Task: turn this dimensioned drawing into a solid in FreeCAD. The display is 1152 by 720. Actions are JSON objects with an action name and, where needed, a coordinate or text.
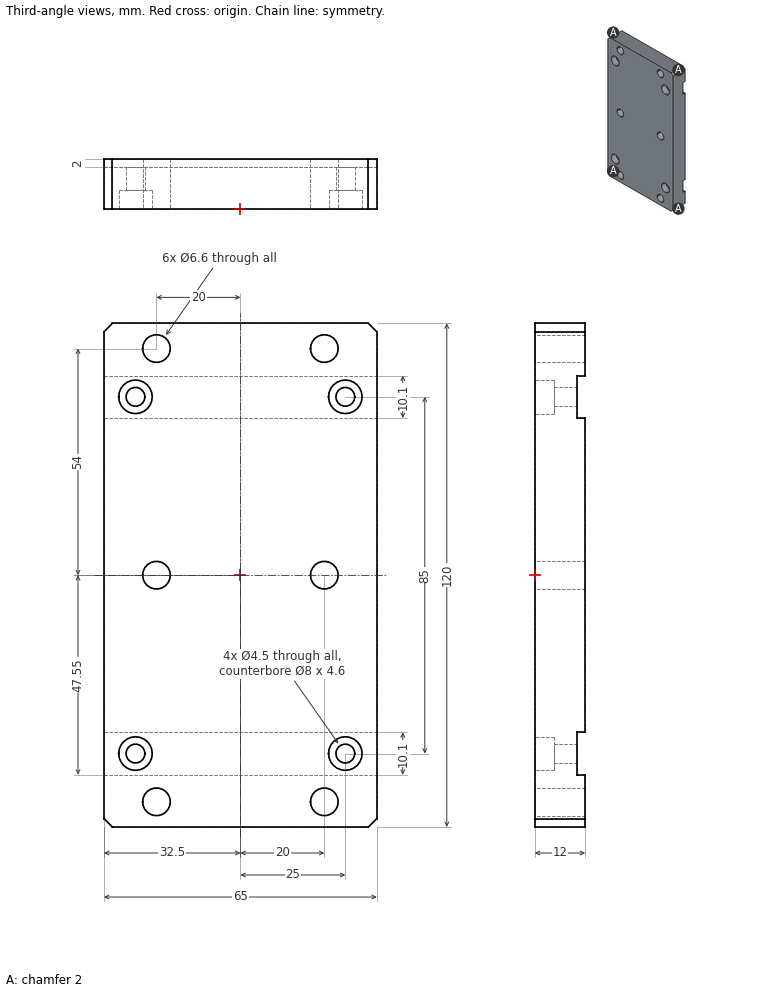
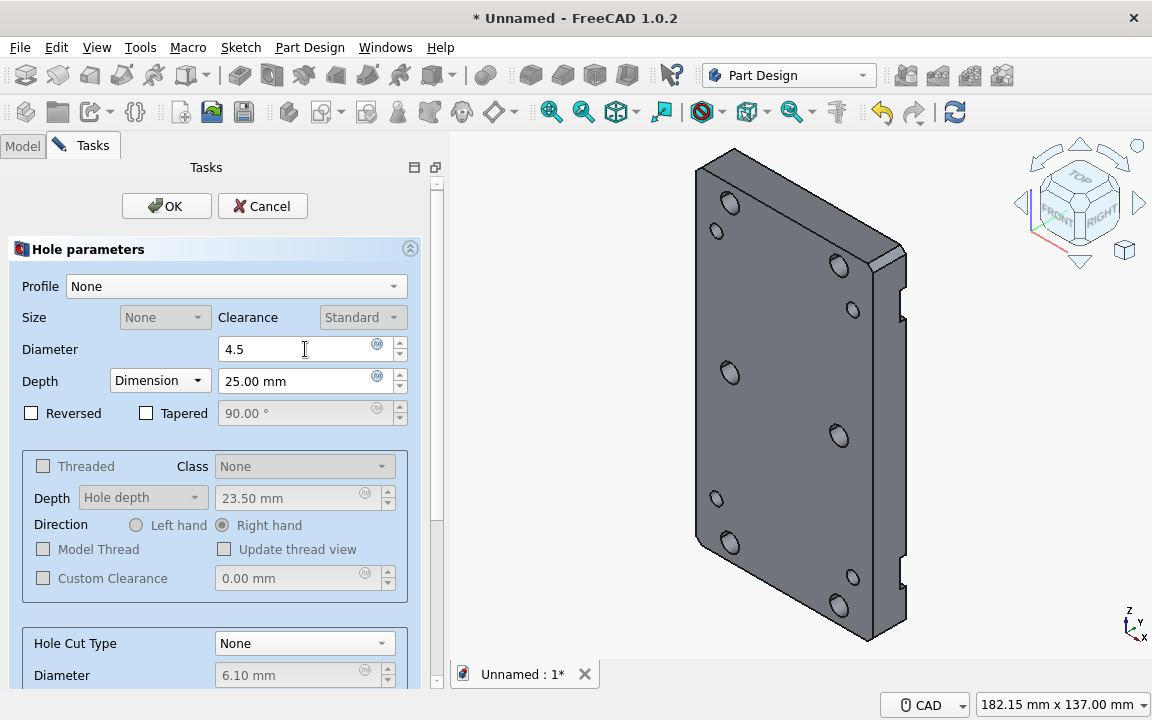
{"action": "left_click", "coordinate": [161, 380]}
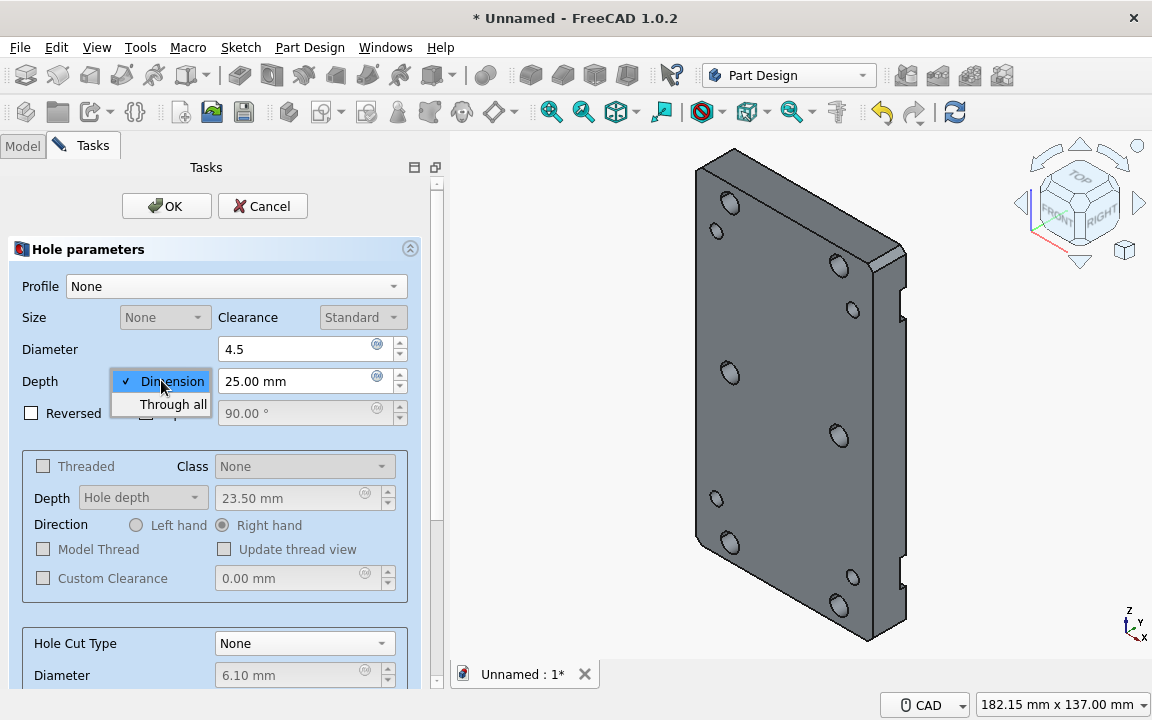
{"action": "left_click", "coordinate": [160, 404]}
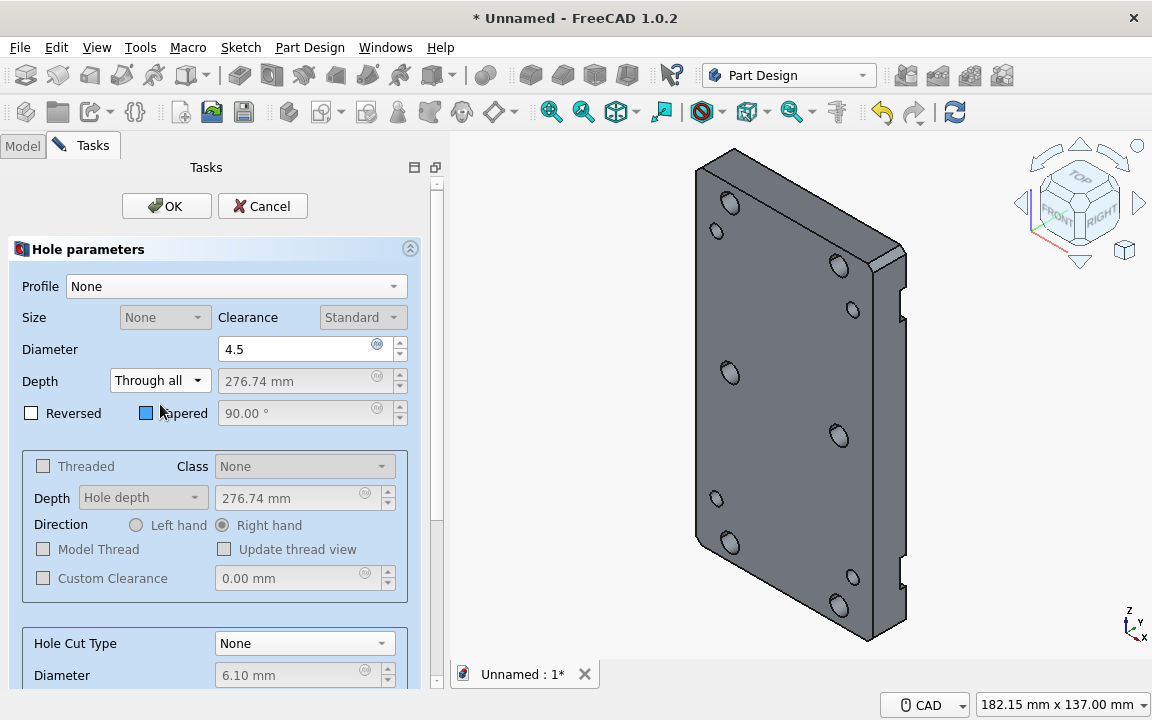
{"action": "left_click", "coordinate": [306, 644]}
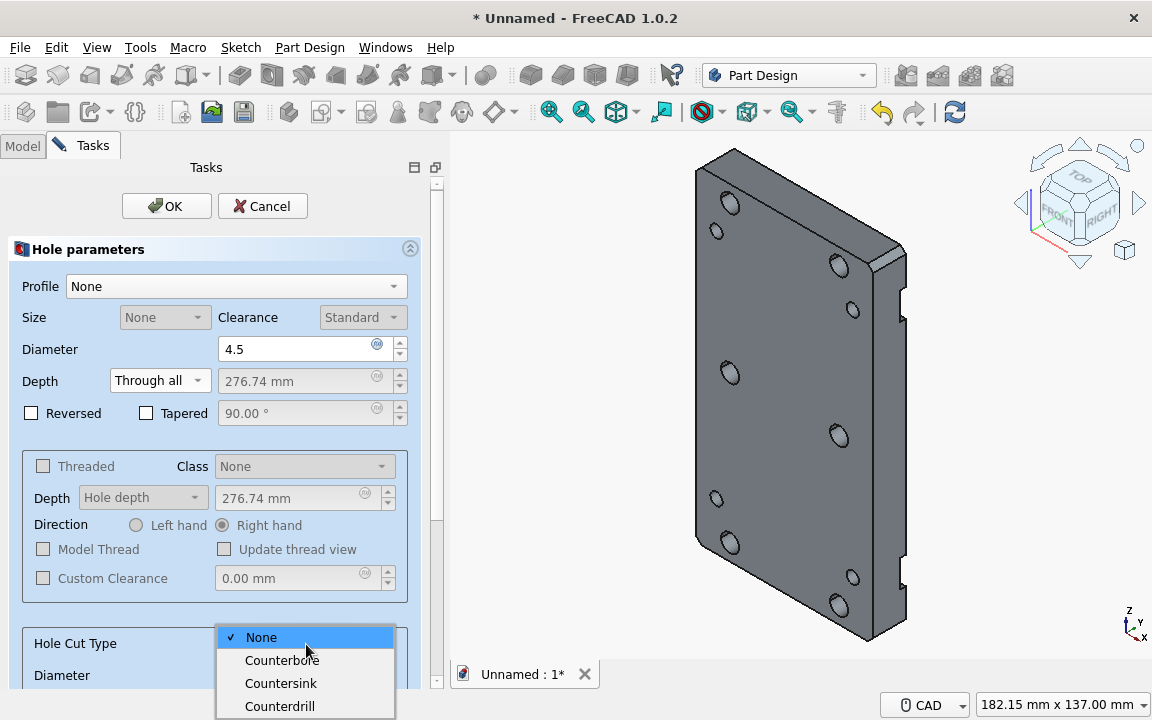
{"action": "left_click", "coordinate": [304, 660]}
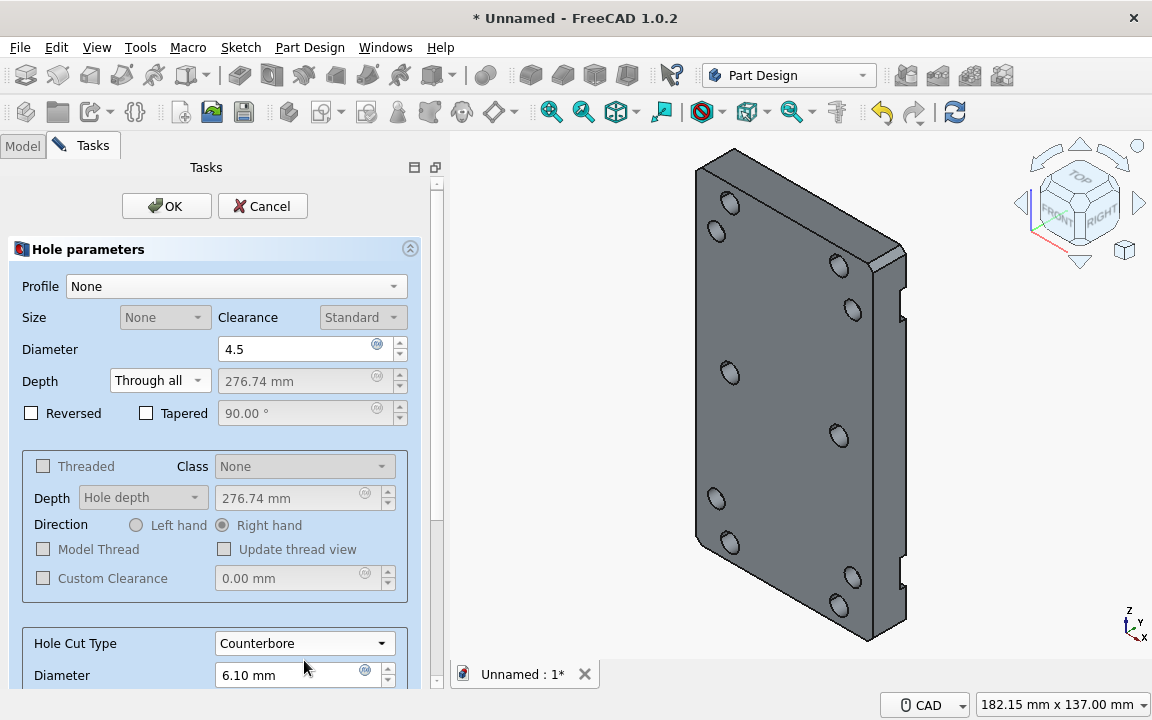
{"action": "triple_click", "coordinate": [298, 675]}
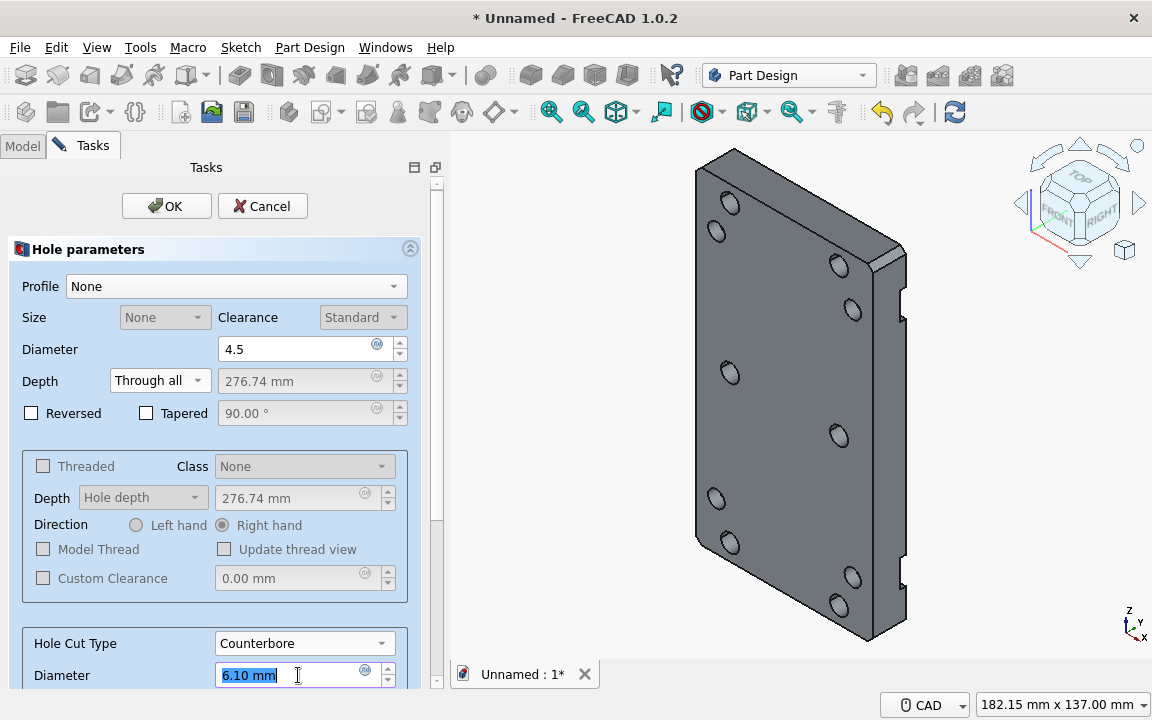
{"action": "type", "text": "8"}
{"action": "key", "text": "Tab"}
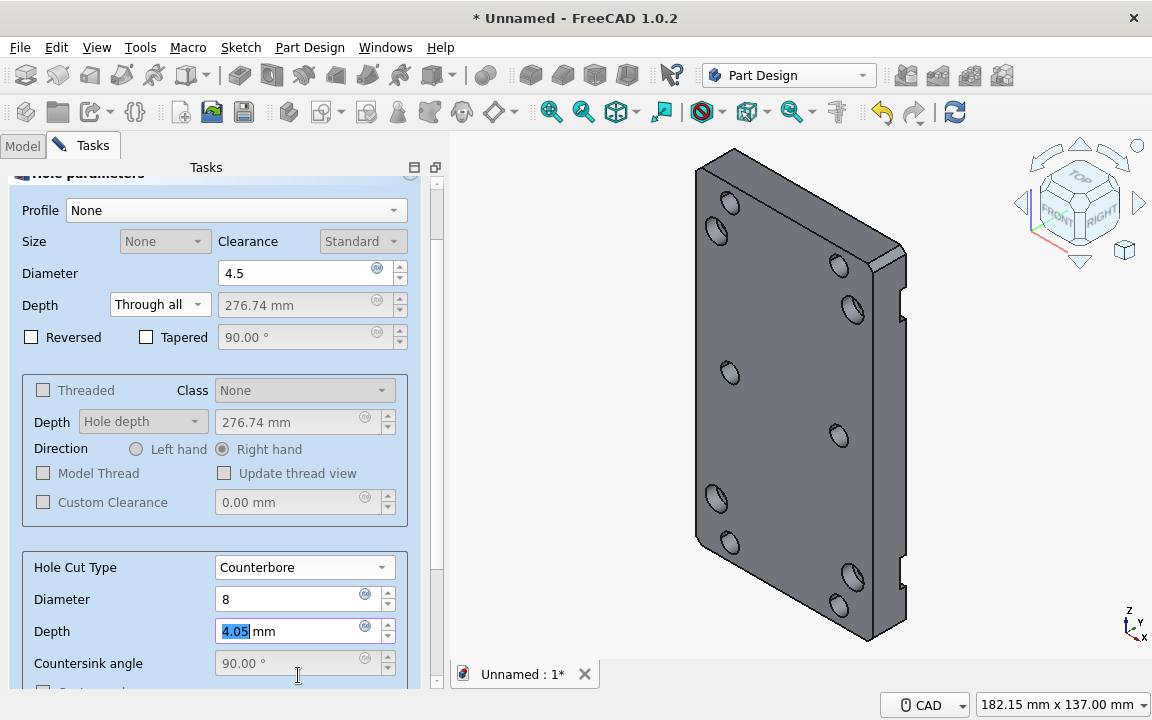
{"action": "type", "text": "4.6"}
{"action": "key", "text": "Tab"}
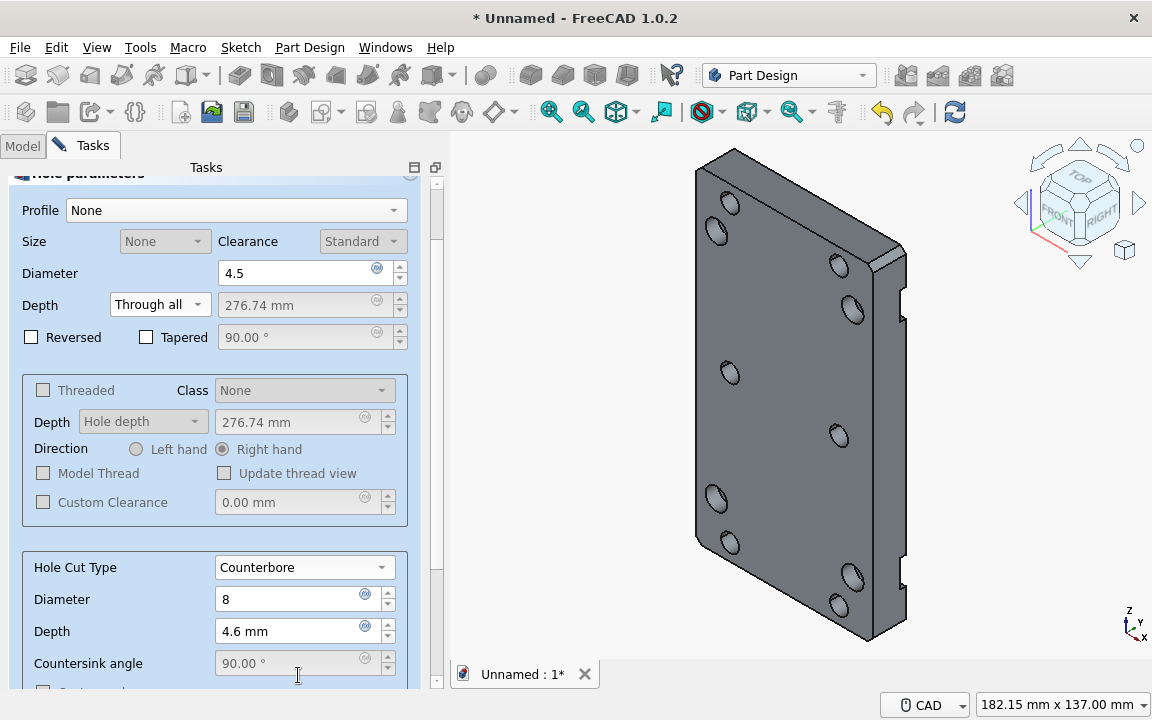
{"action": "scroll", "coordinate": [437, 432], "scroll_direction": "up", "scroll_amount": 3}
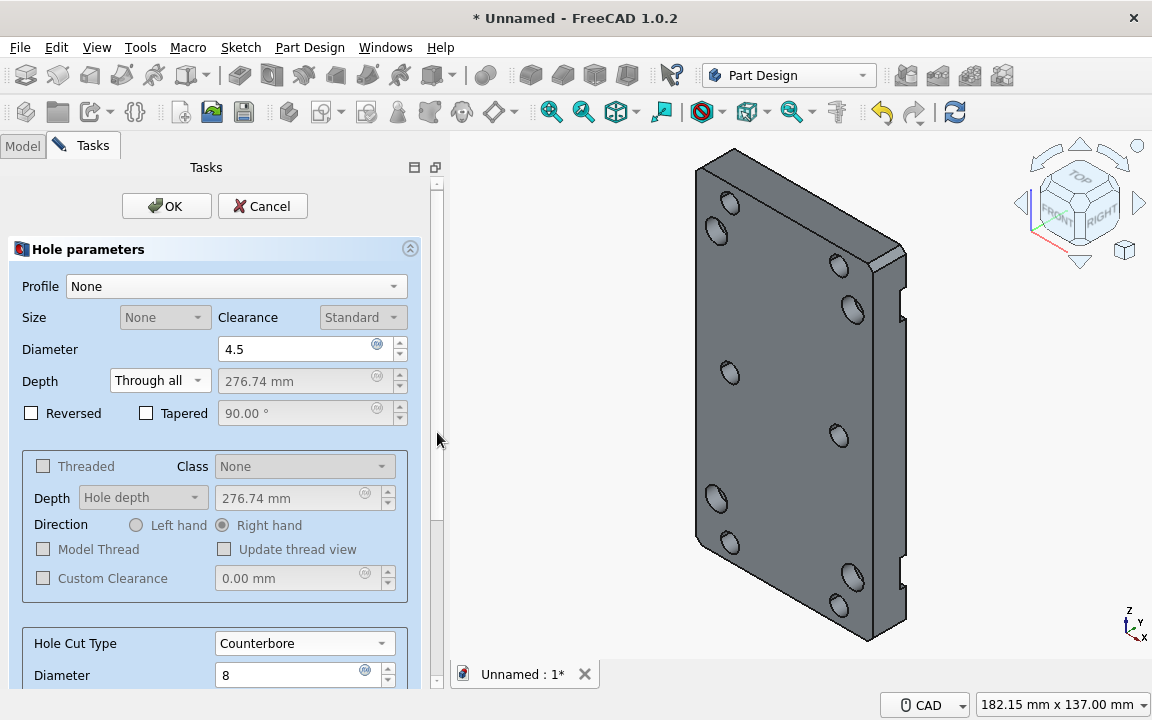
{"action": "left_click", "coordinate": [167, 206]}